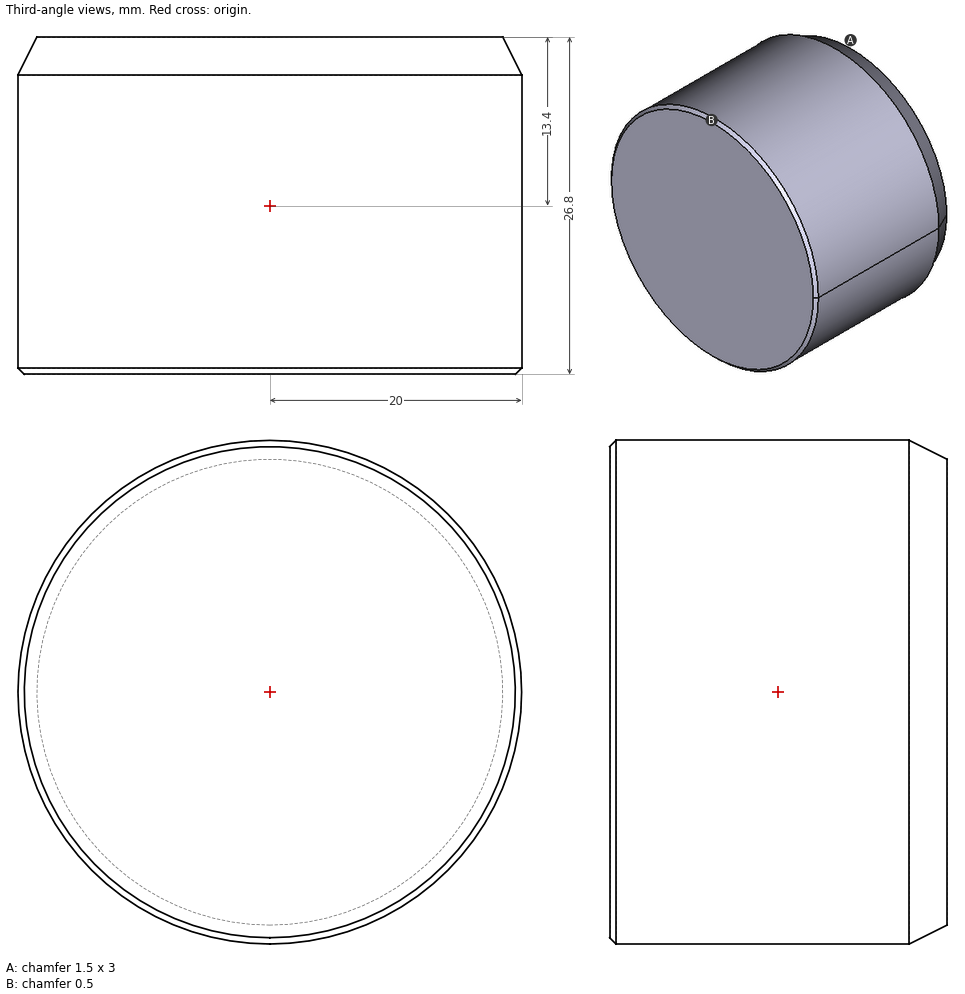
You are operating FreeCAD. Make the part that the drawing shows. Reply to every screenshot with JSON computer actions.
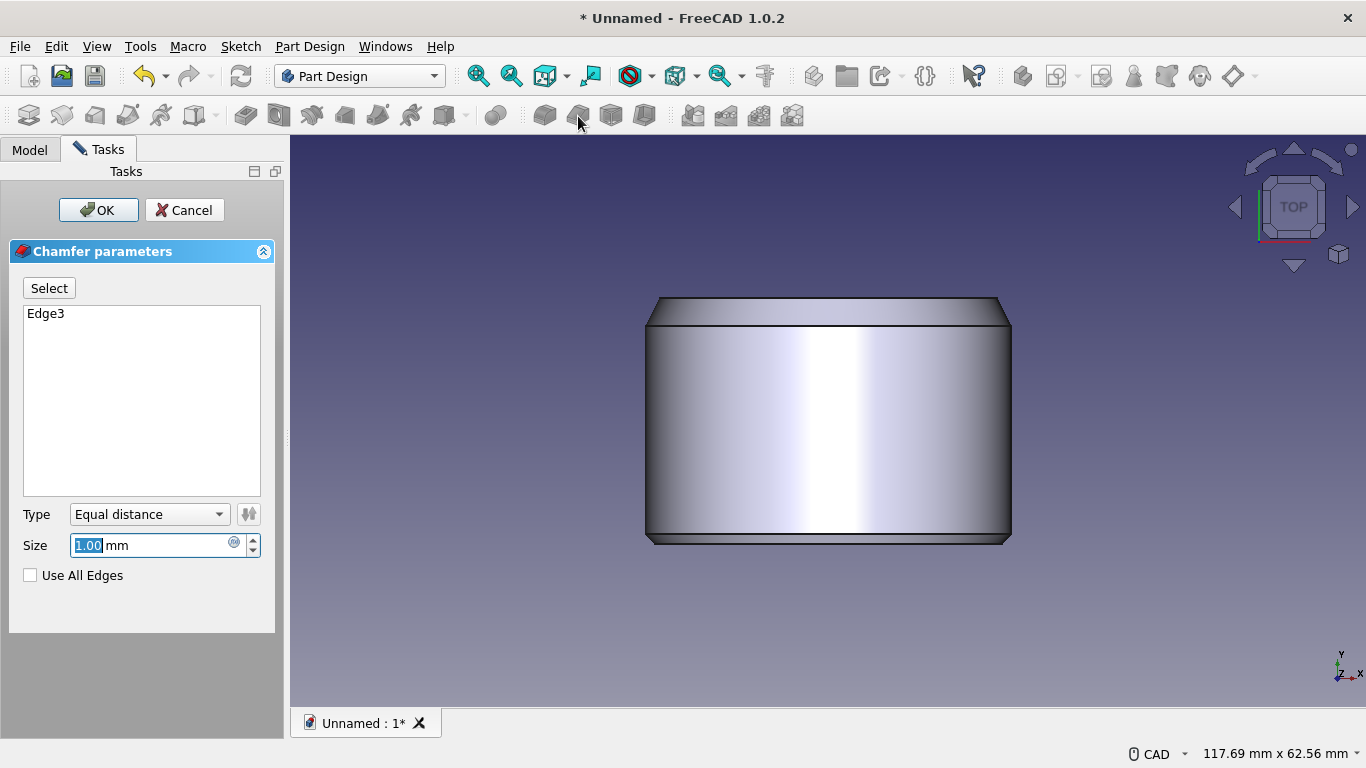
{"action": "type", "text": "0.5"}
{"action": "key", "text": "Tab"}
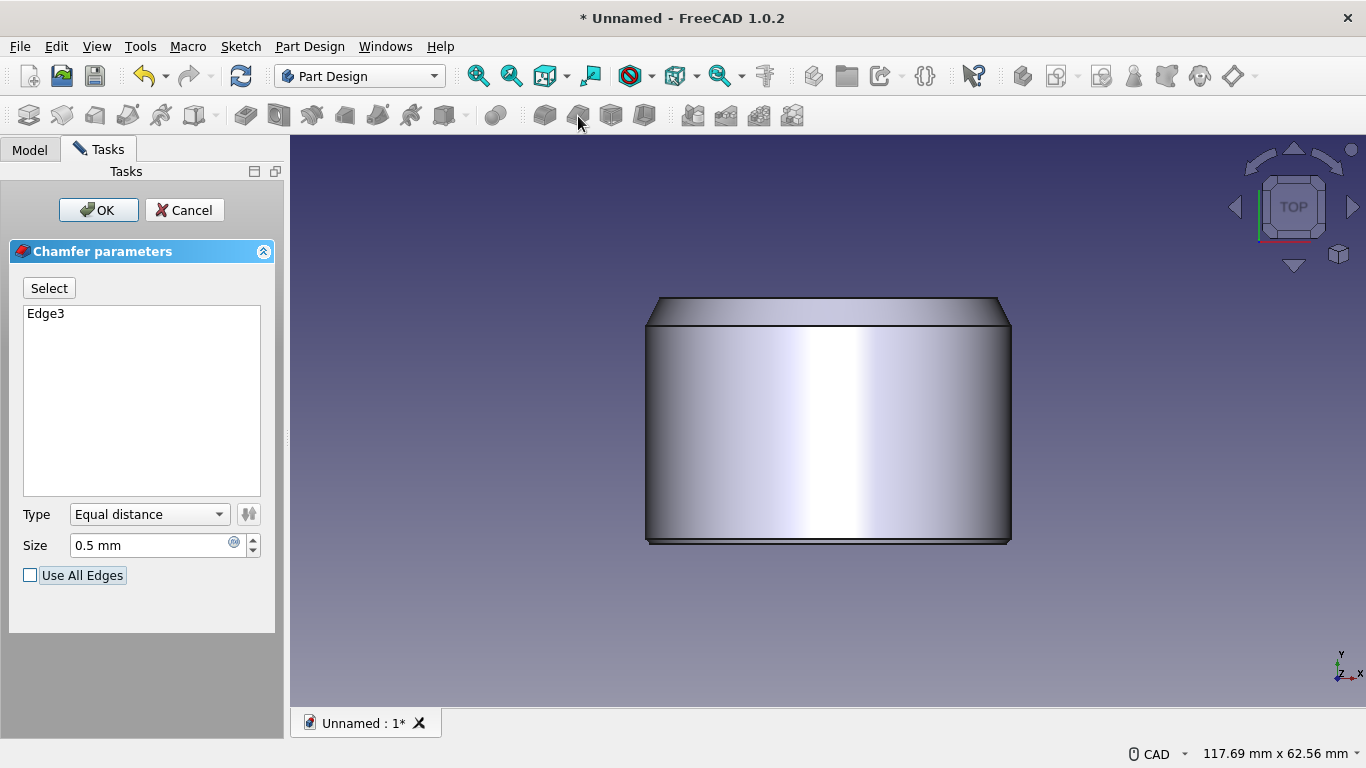
{"action": "left_click", "coordinate": [99, 210]}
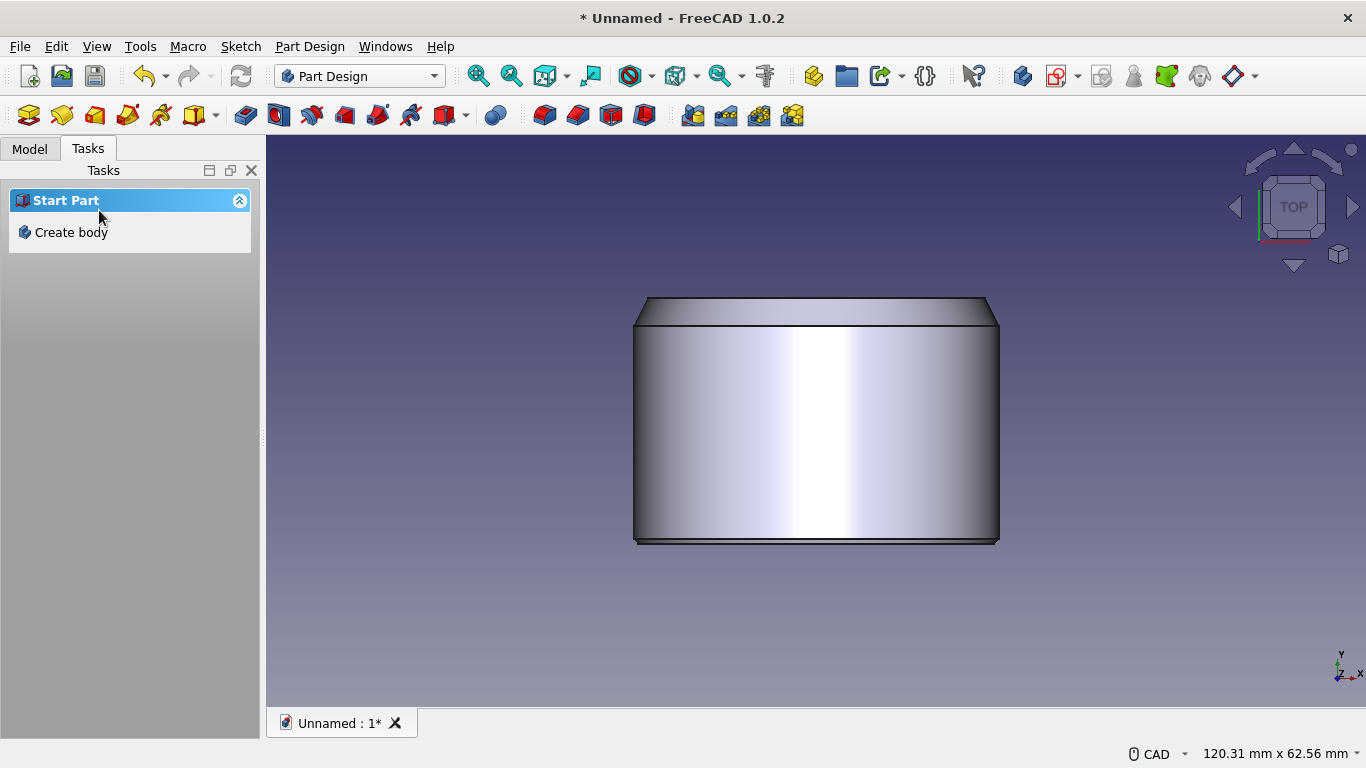
{"action": "key", "text": "0"}